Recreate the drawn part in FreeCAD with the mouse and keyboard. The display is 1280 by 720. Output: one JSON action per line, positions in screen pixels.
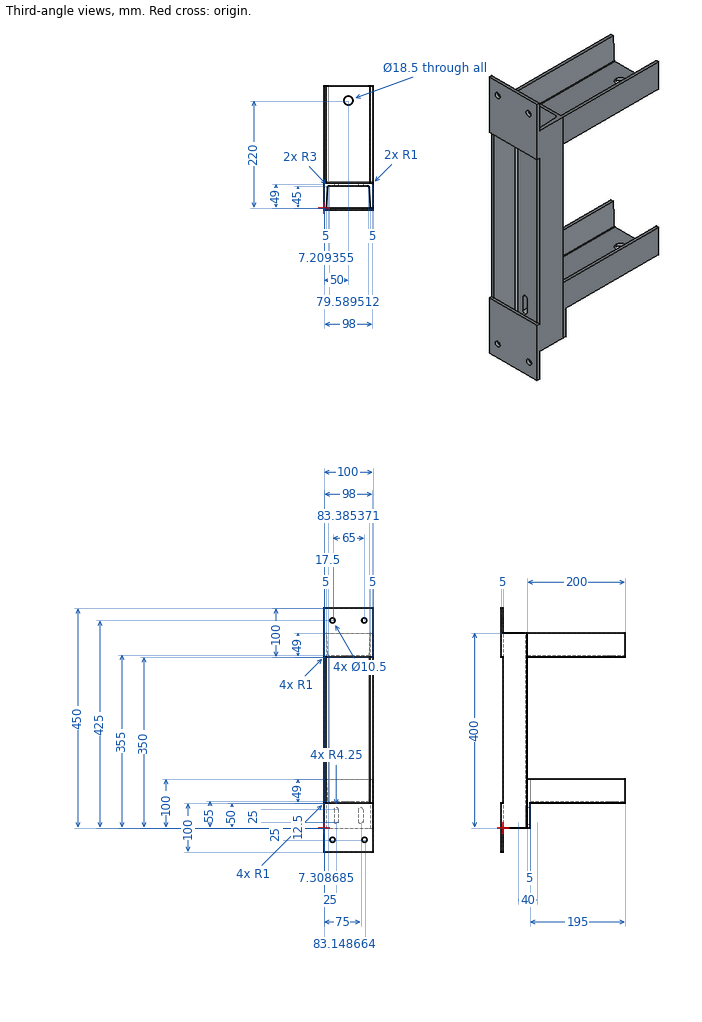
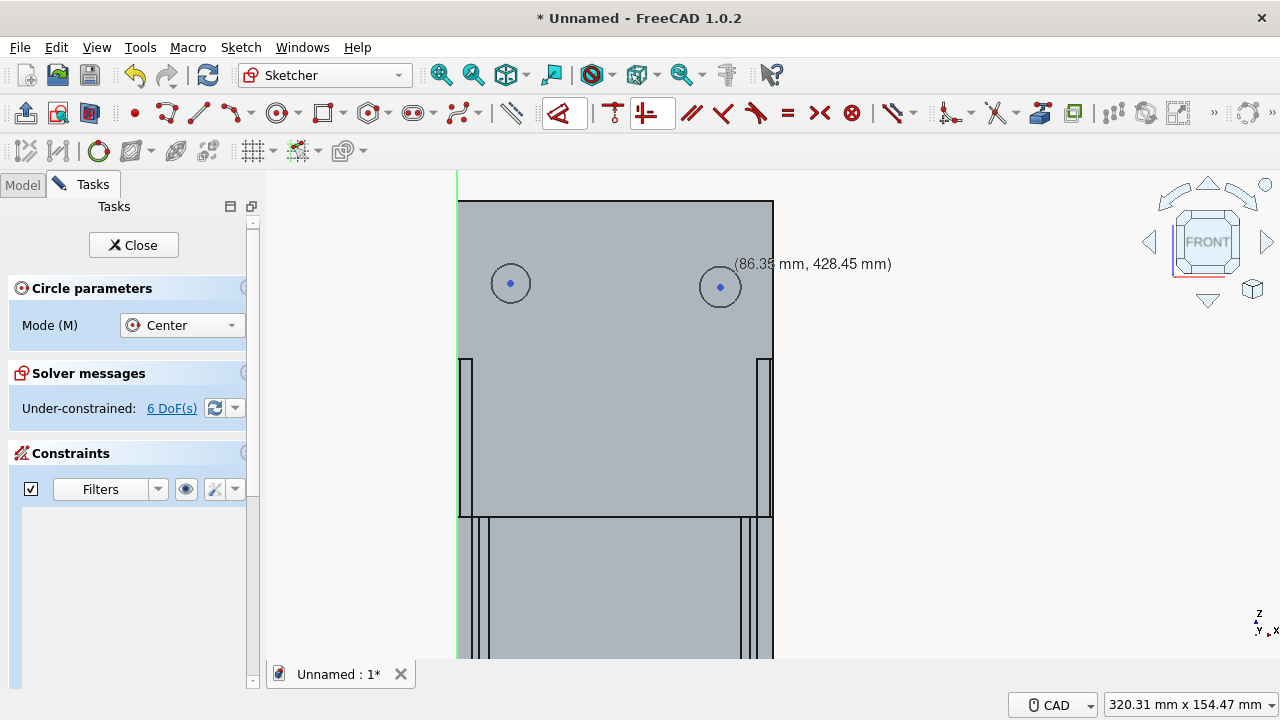
{"action": "scroll", "coordinate": [732, 268], "scroll_direction": "down", "scroll_amount": 8}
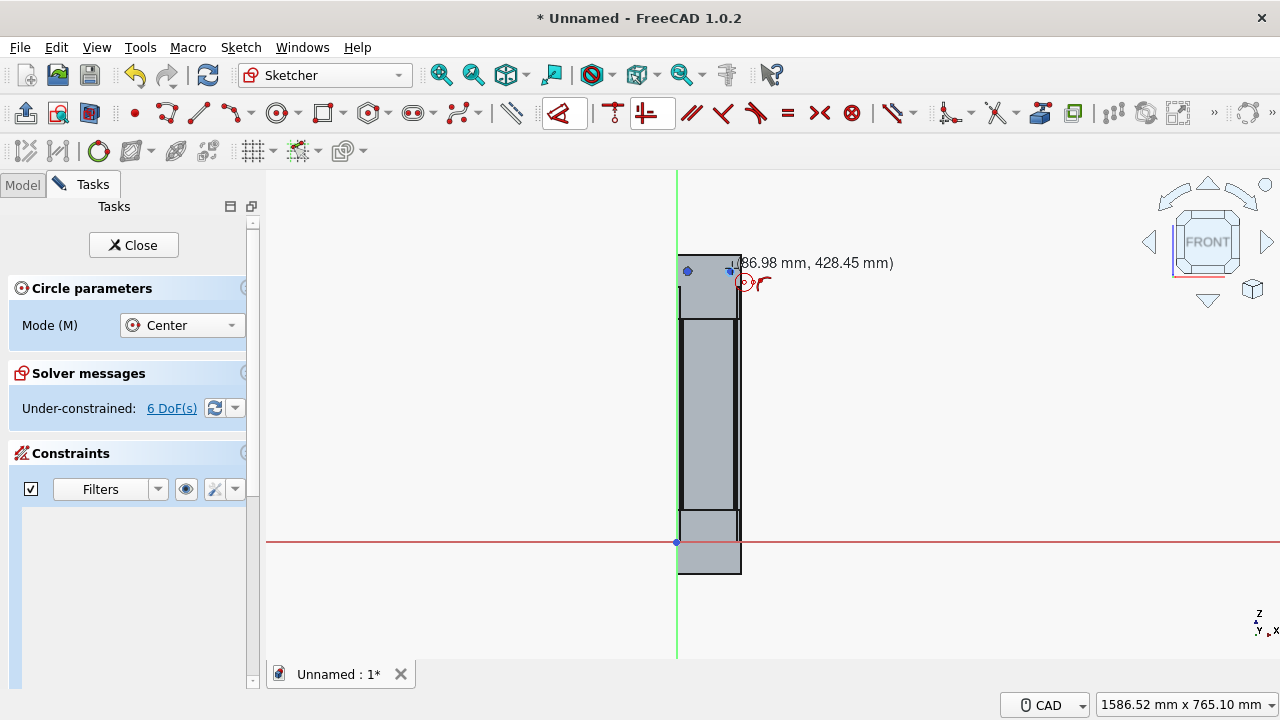
{"action": "scroll", "coordinate": [730, 558], "scroll_direction": "up", "scroll_amount": 10}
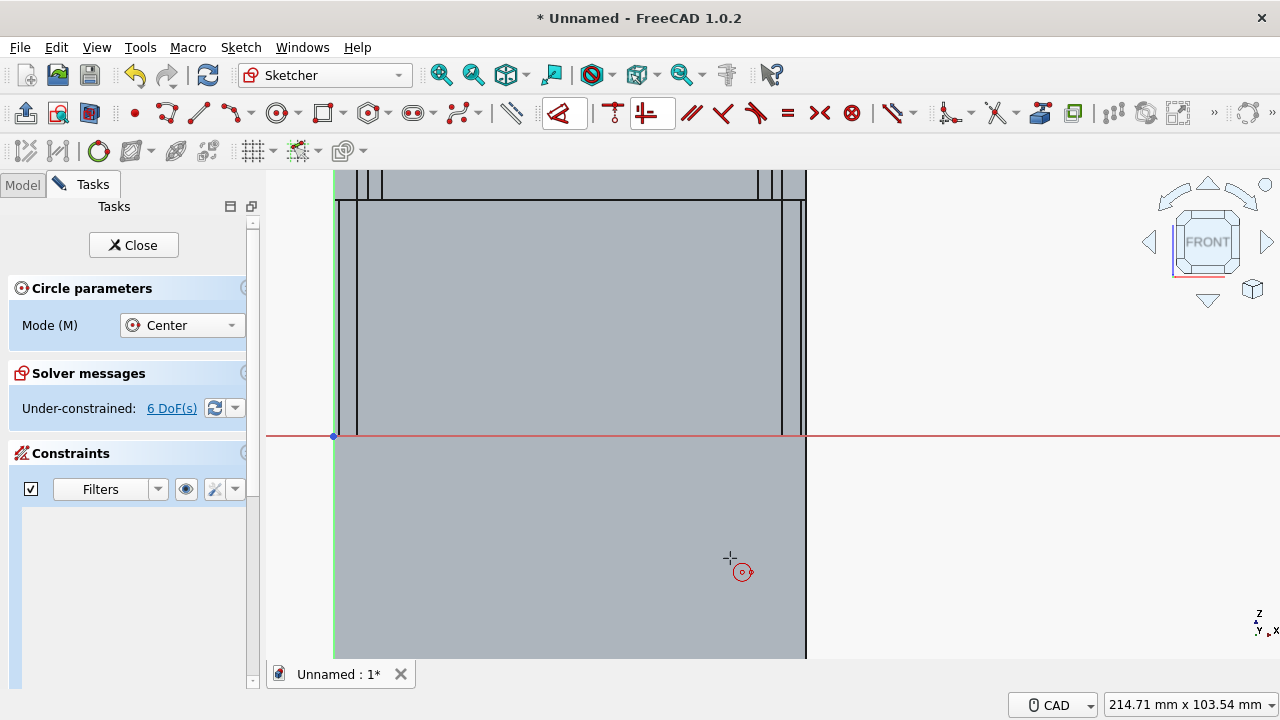
{"action": "scroll", "coordinate": [730, 559], "scroll_direction": "down", "scroll_amount": 10}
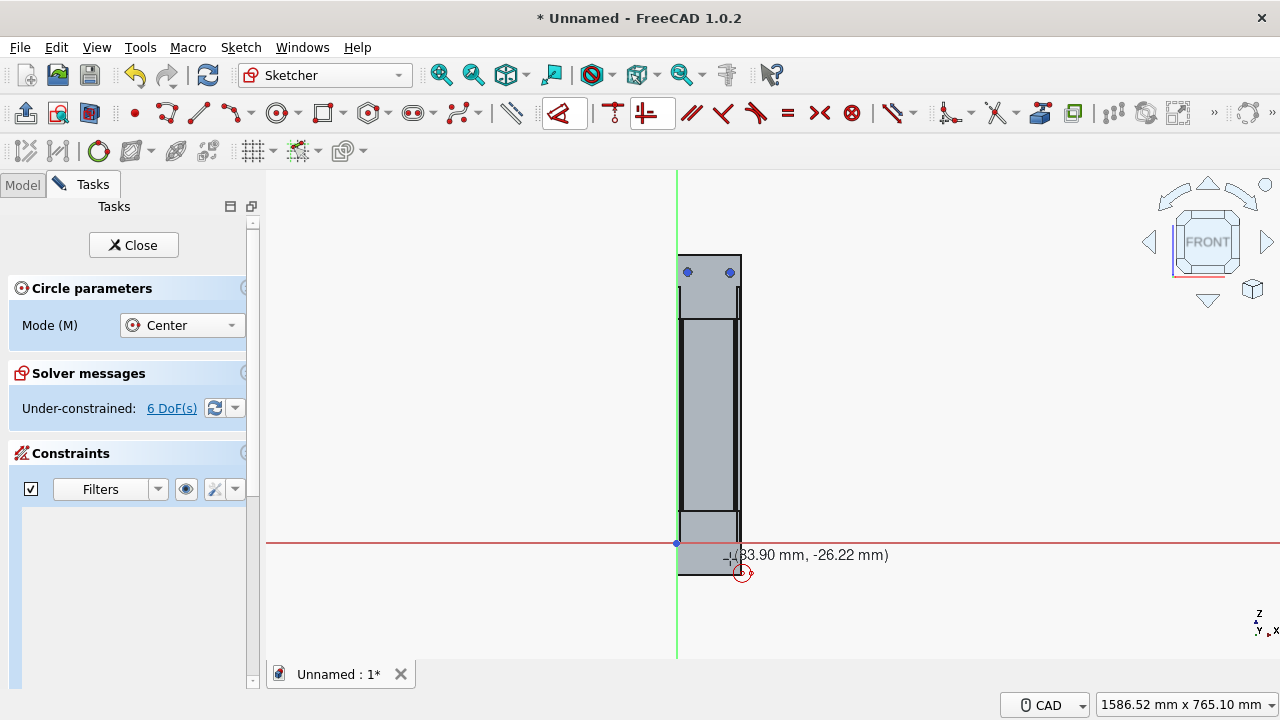
{"action": "left_click", "coordinate": [730, 559]}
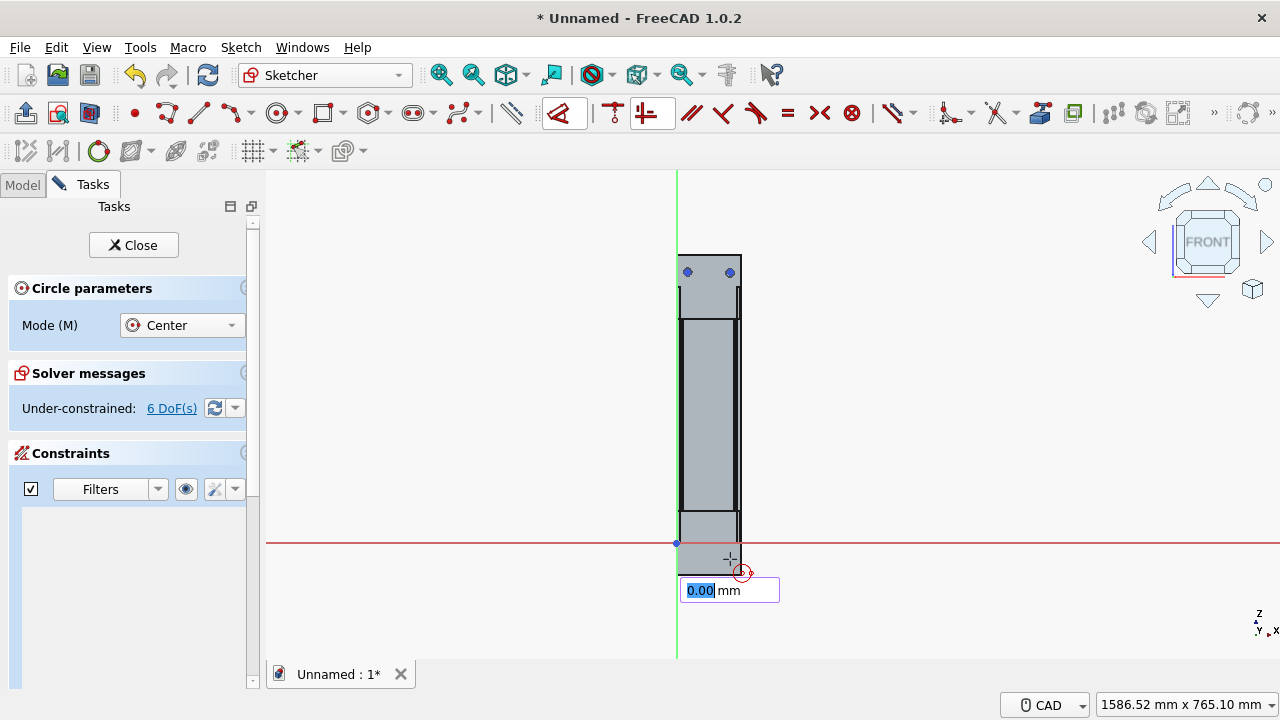
{"action": "scroll", "coordinate": [732, 561], "scroll_direction": "up", "scroll_amount": 8}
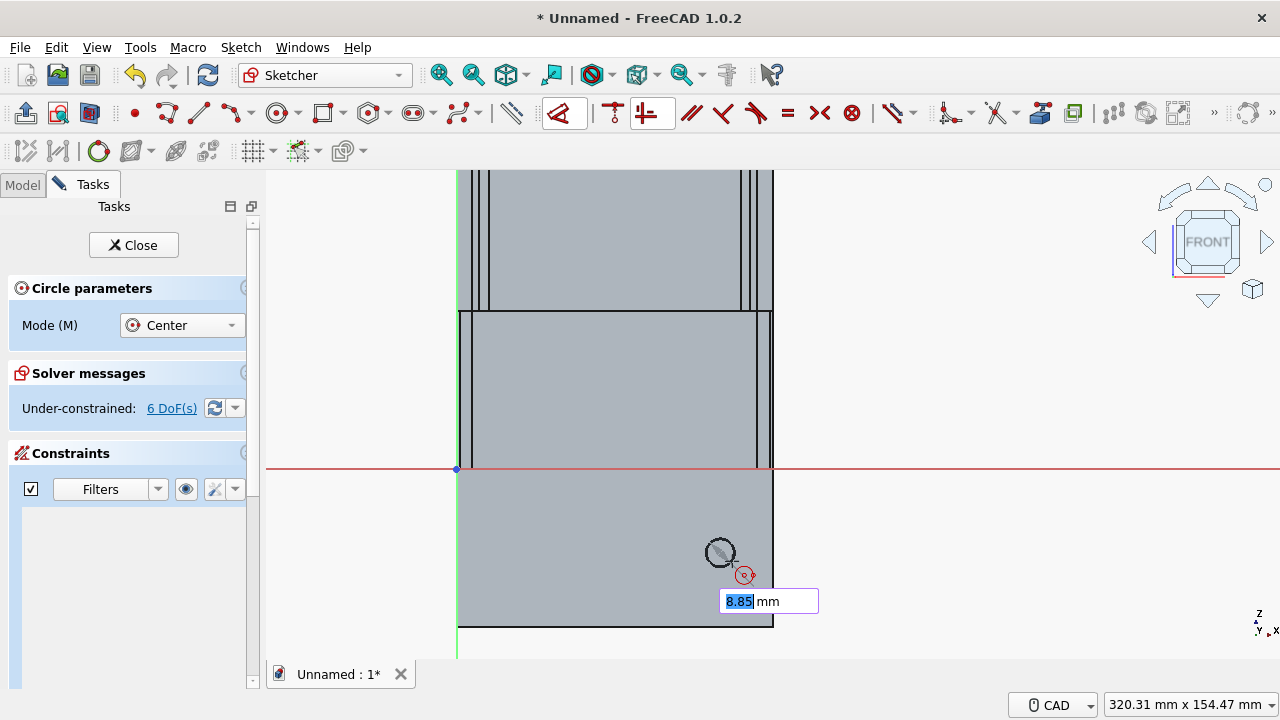
{"action": "left_click", "coordinate": [732, 560]}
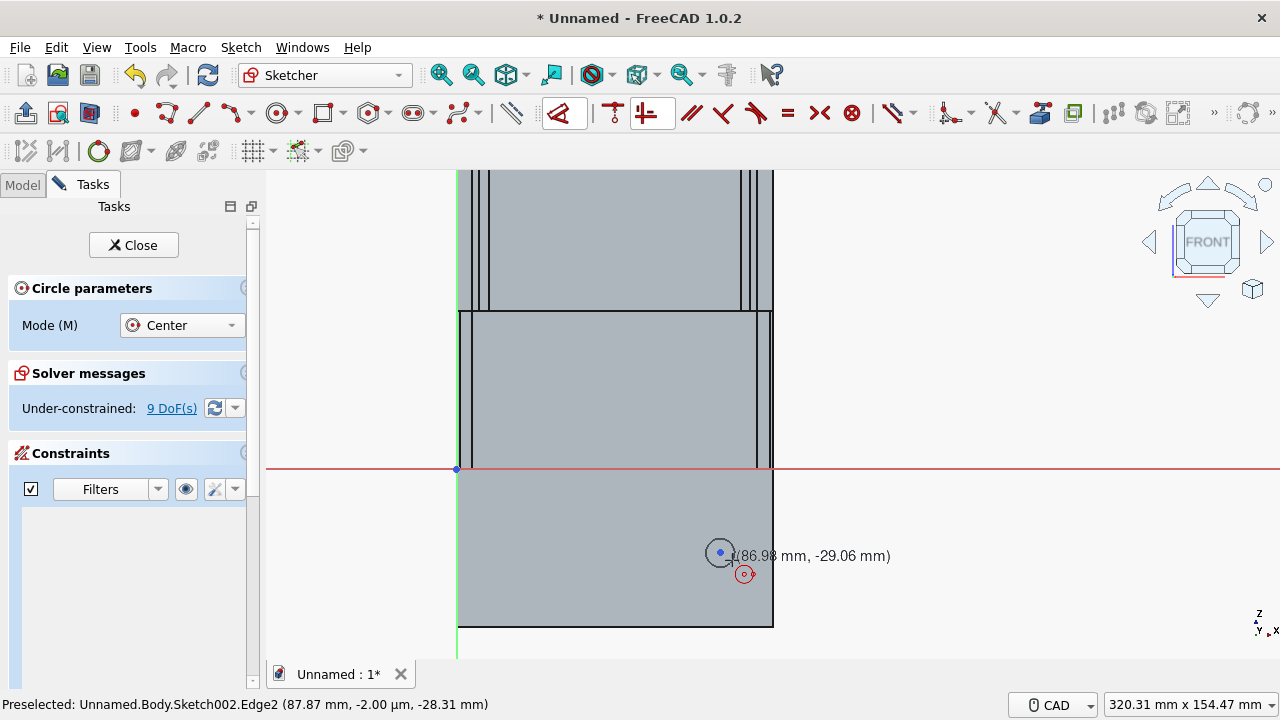
{"action": "scroll", "coordinate": [512, 548], "scroll_direction": "up", "scroll_amount": 2}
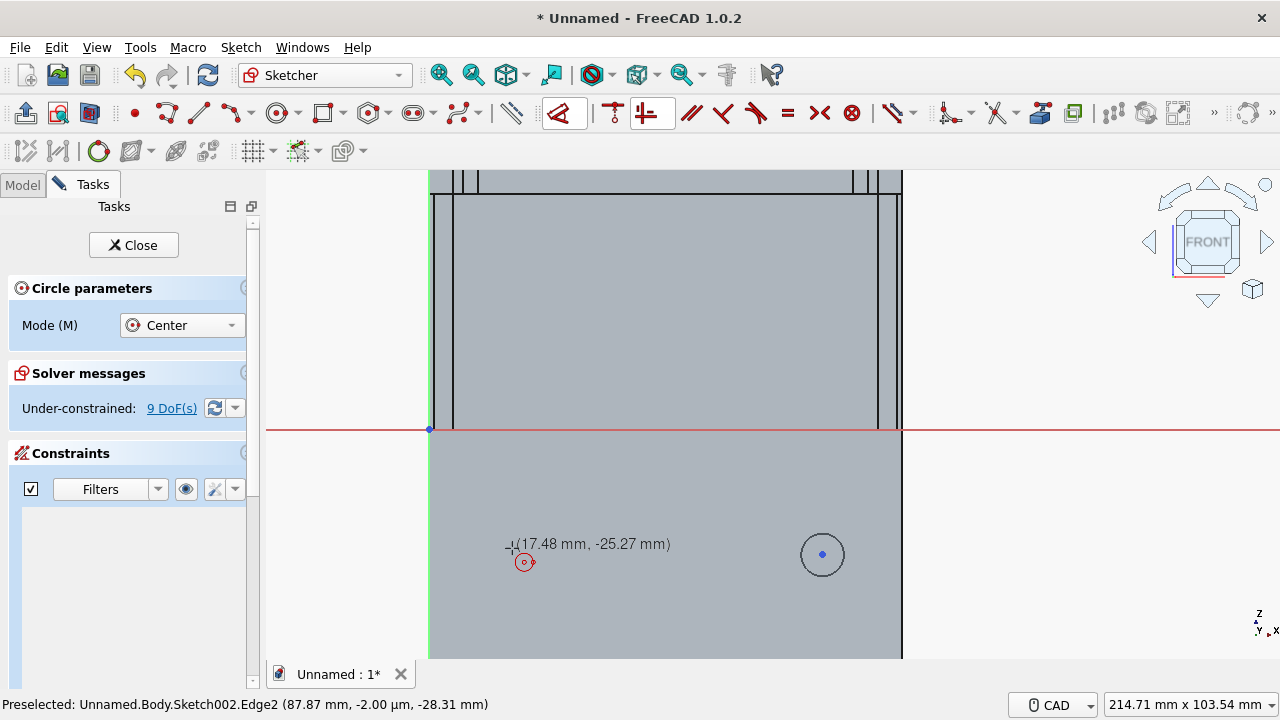
{"action": "scroll", "coordinate": [715, 560], "scroll_direction": "down", "scroll_amount": 10}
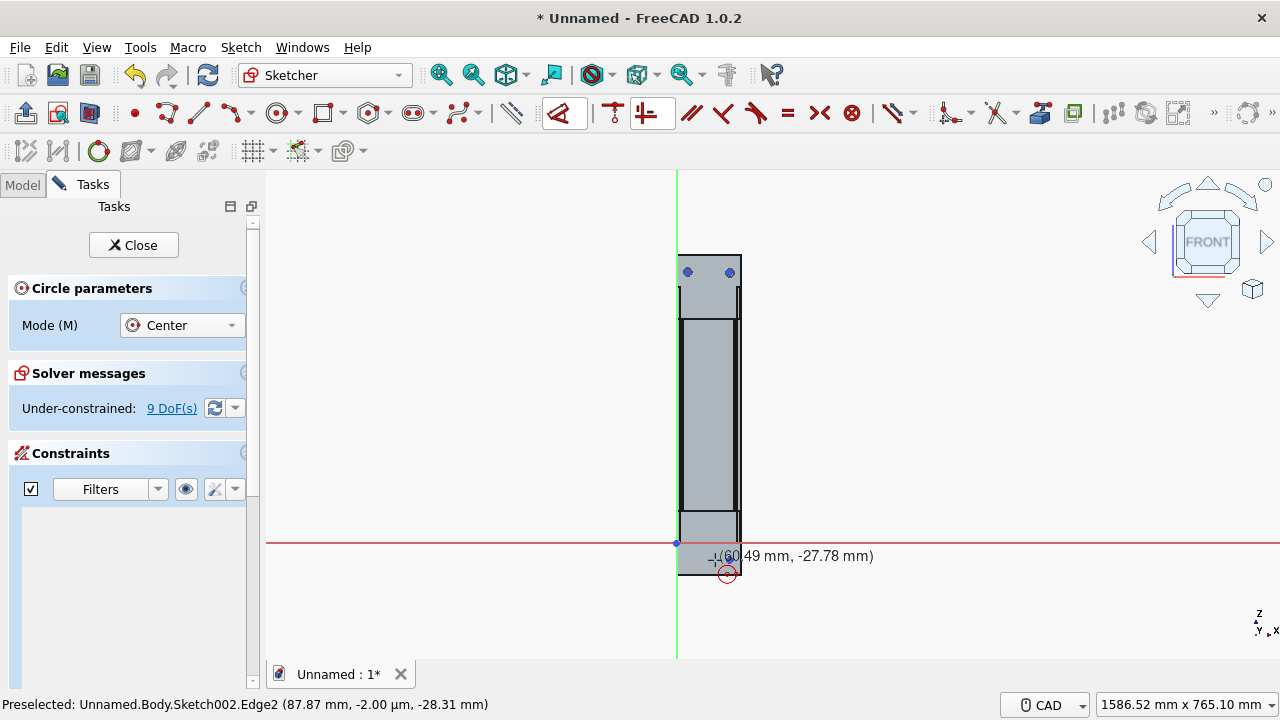
{"action": "scroll", "coordinate": [688, 559], "scroll_direction": "up", "scroll_amount": 2}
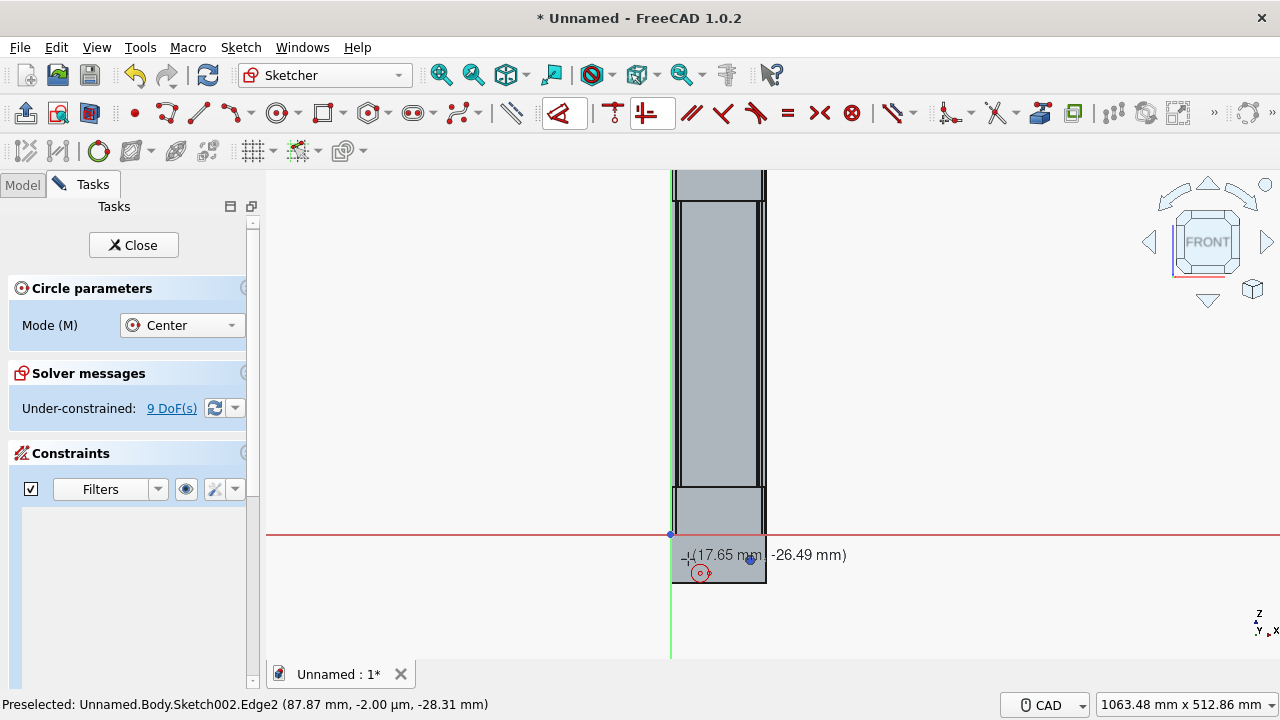
{"action": "left_click", "coordinate": [688, 559]}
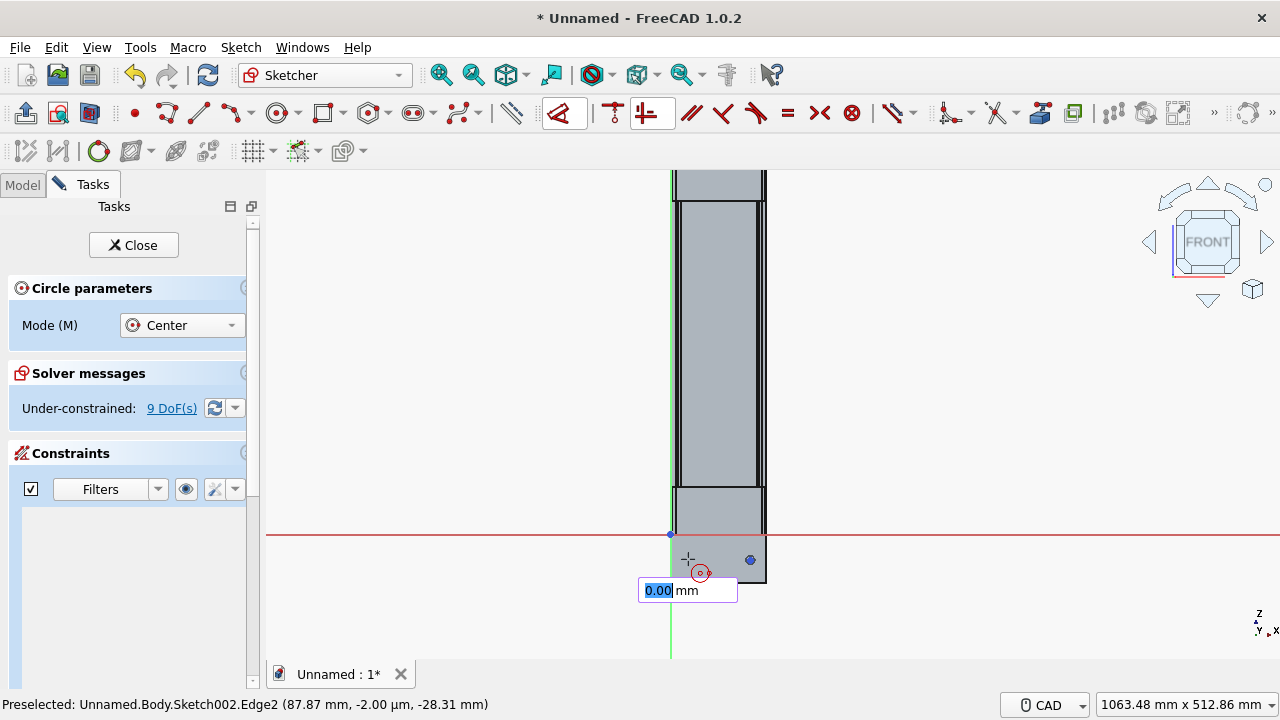
{"action": "scroll", "coordinate": [691, 555], "scroll_direction": "up", "scroll_amount": 6}